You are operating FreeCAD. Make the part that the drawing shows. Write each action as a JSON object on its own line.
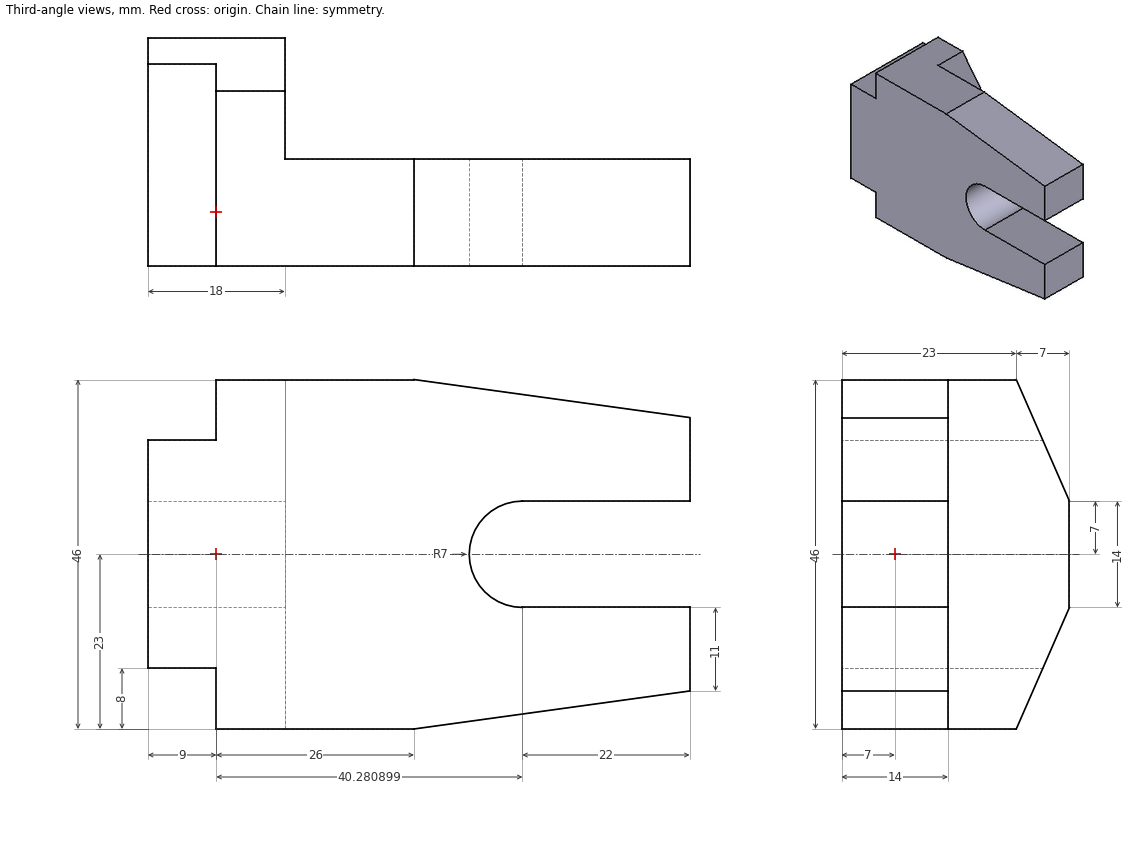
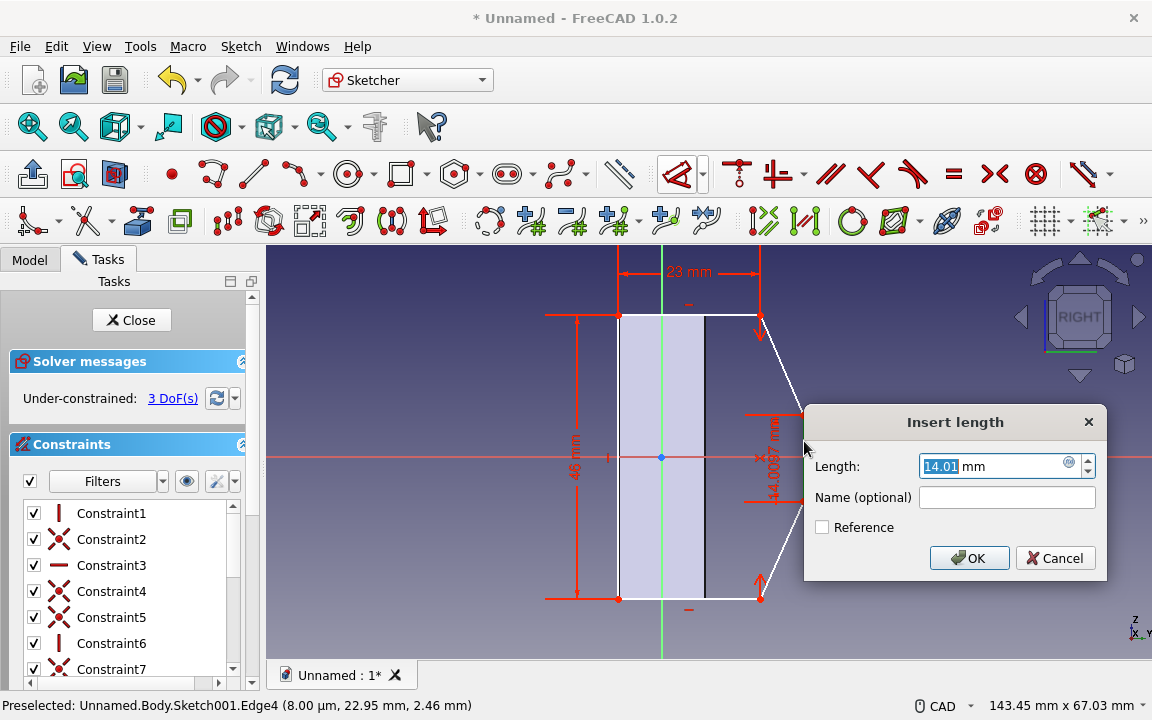
{"action": "type", "text": "14"}
{"action": "key", "text": "Return"}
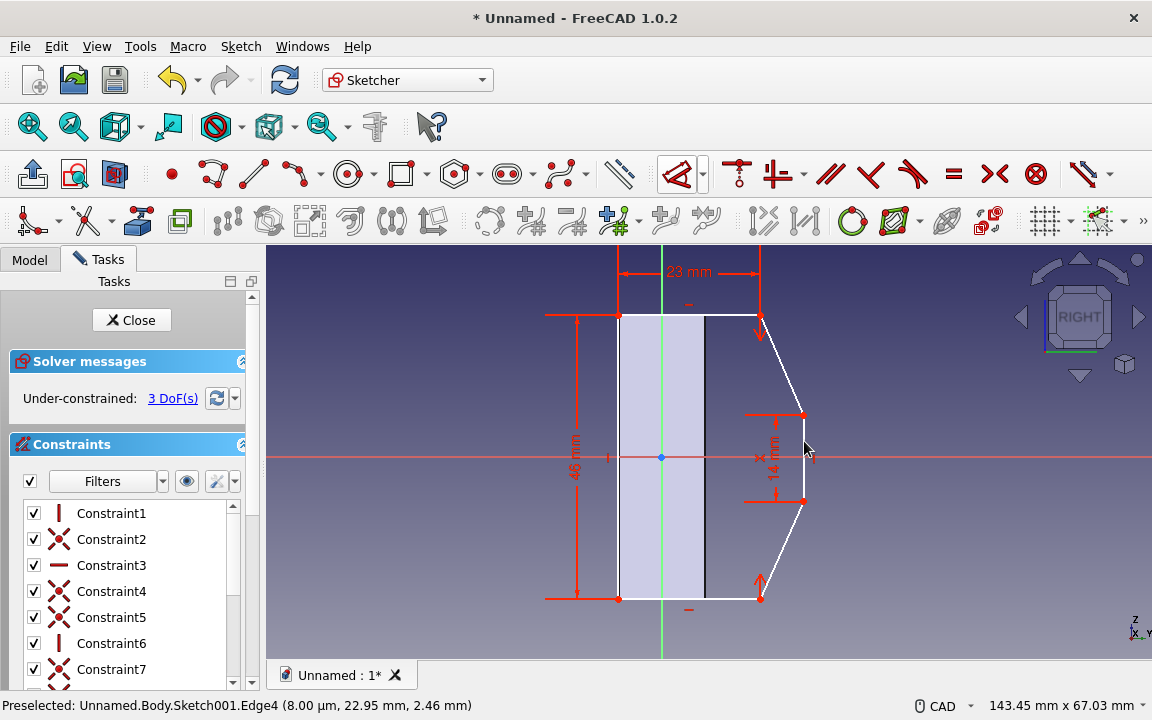
{"action": "left_click", "coordinate": [618, 599]}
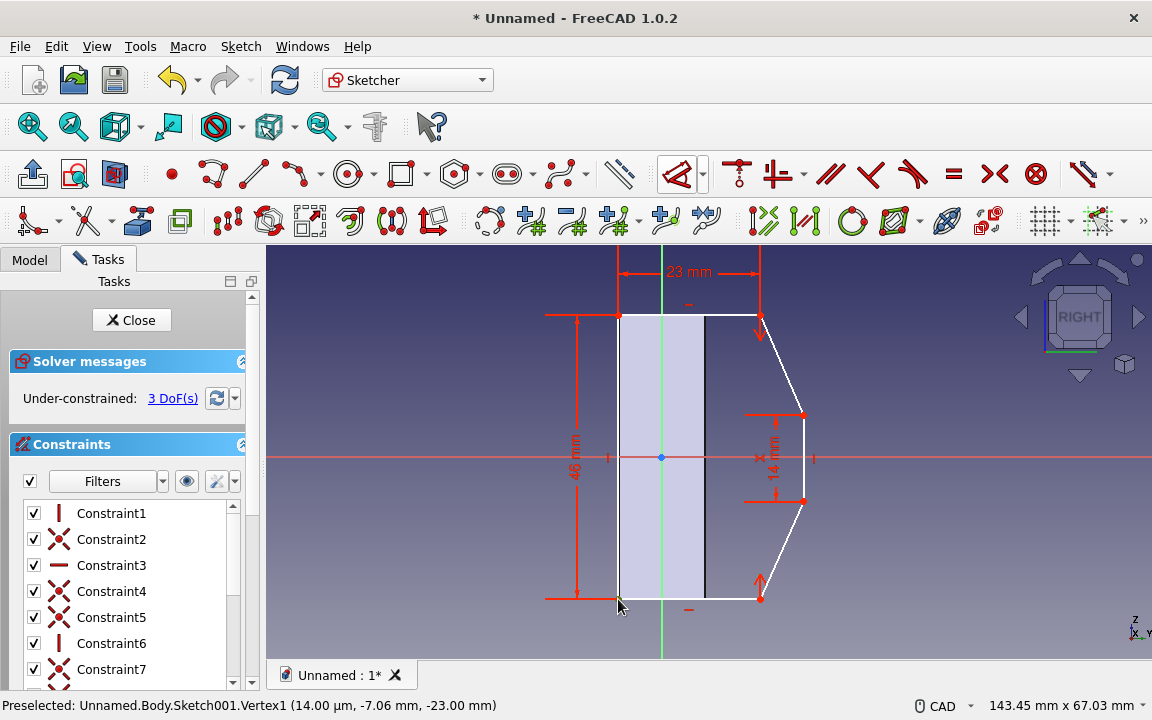
{"action": "key", "text": "l"}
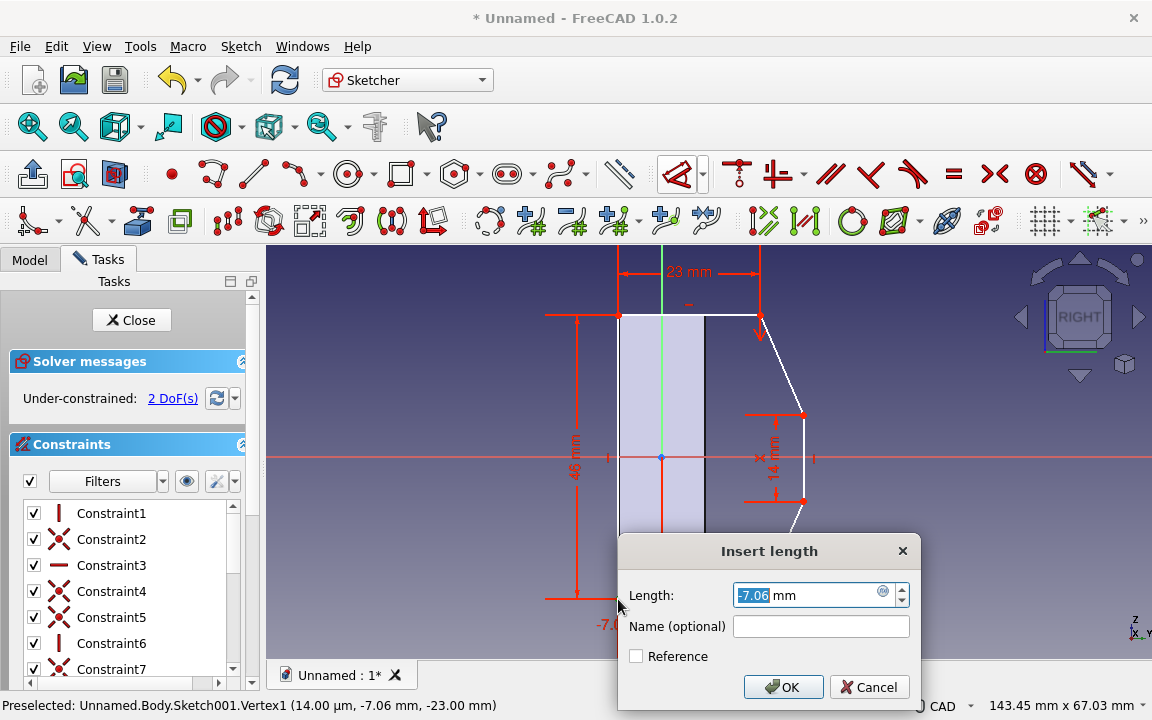
{"action": "type", "text": "-7"}
{"action": "key", "text": "Return"}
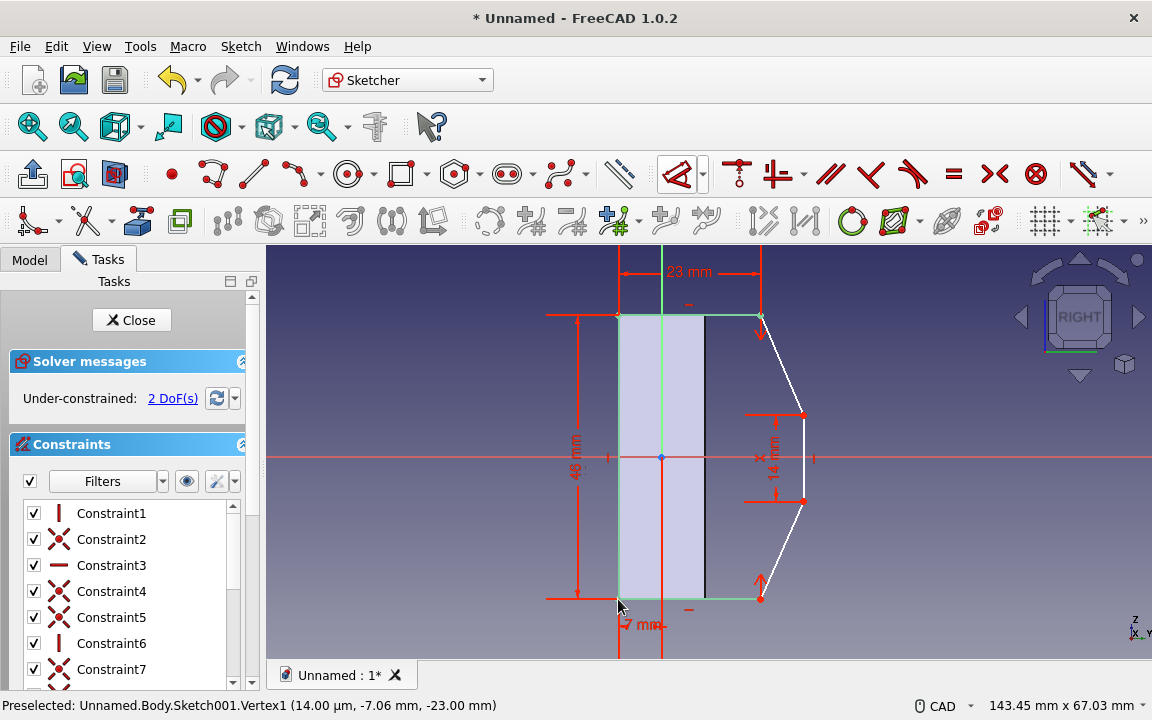
{"action": "left_click", "coordinate": [804, 415]}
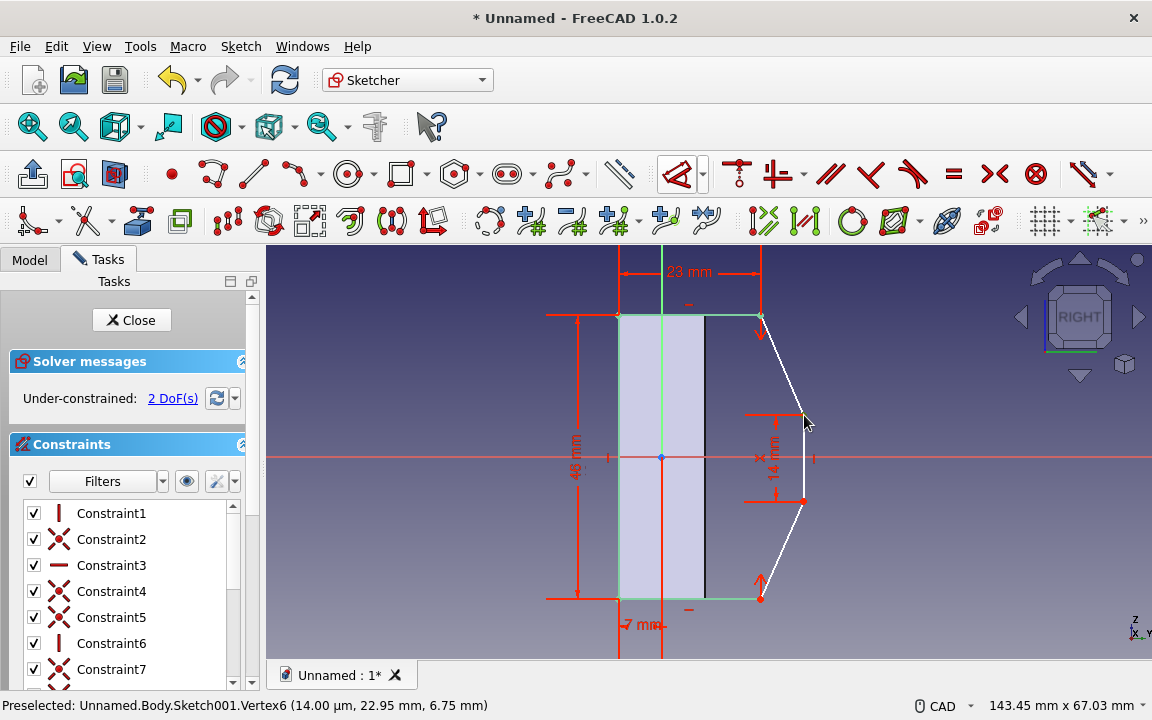
{"action": "key", "text": "i"}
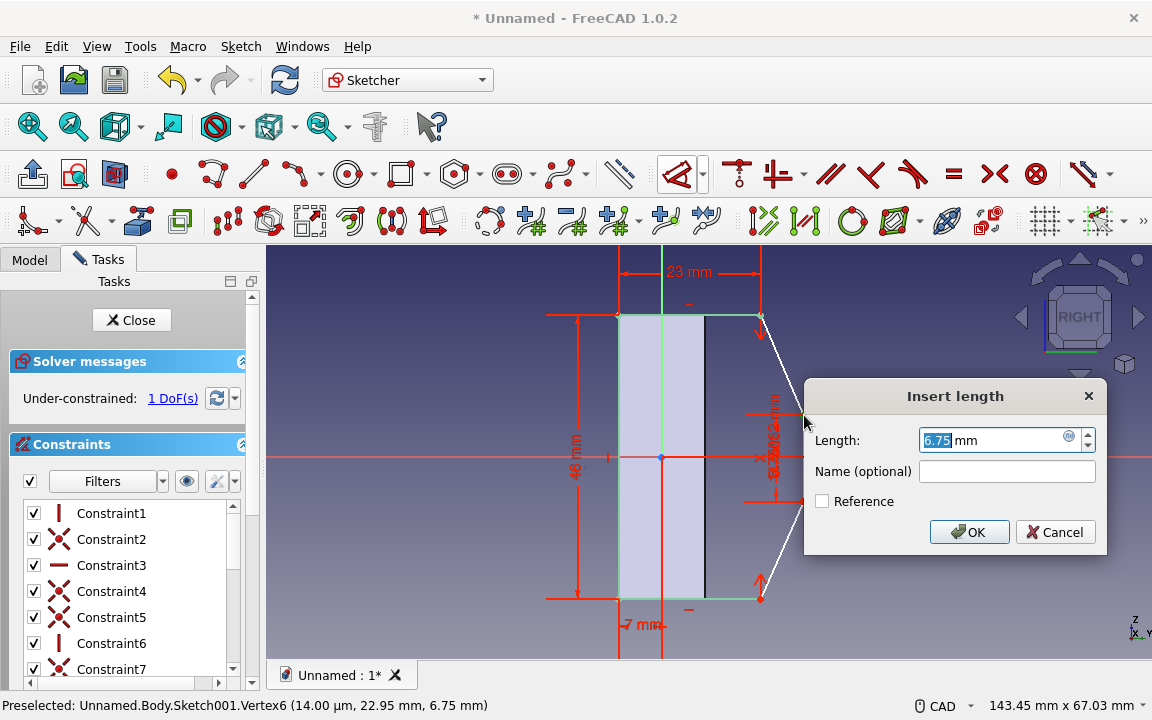
{"action": "type", "text": "7"}
{"action": "key", "text": "Return"}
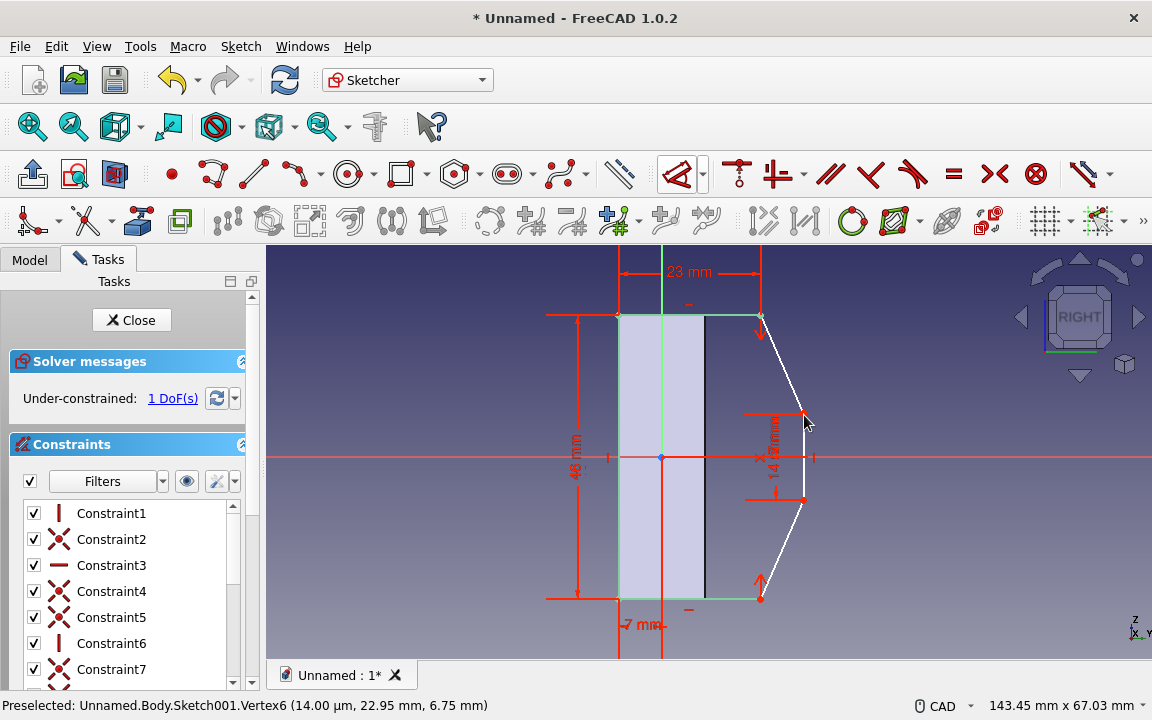
{"action": "left_click", "coordinate": [774, 345]}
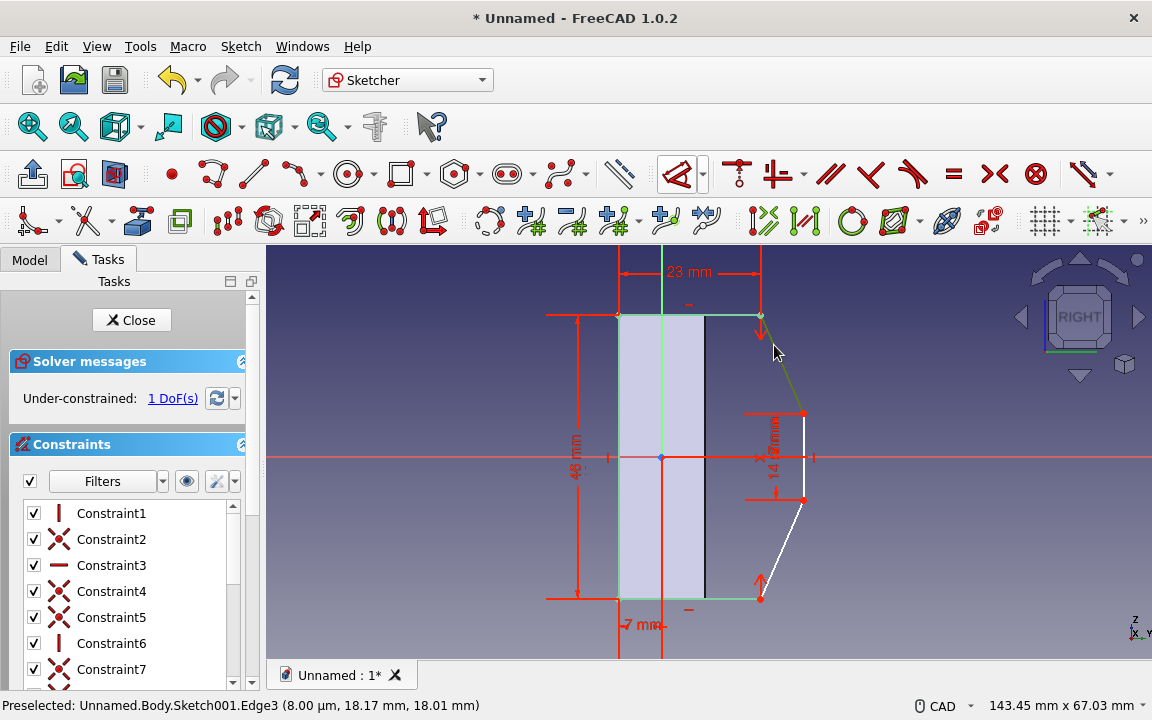
{"action": "key", "text": "l"}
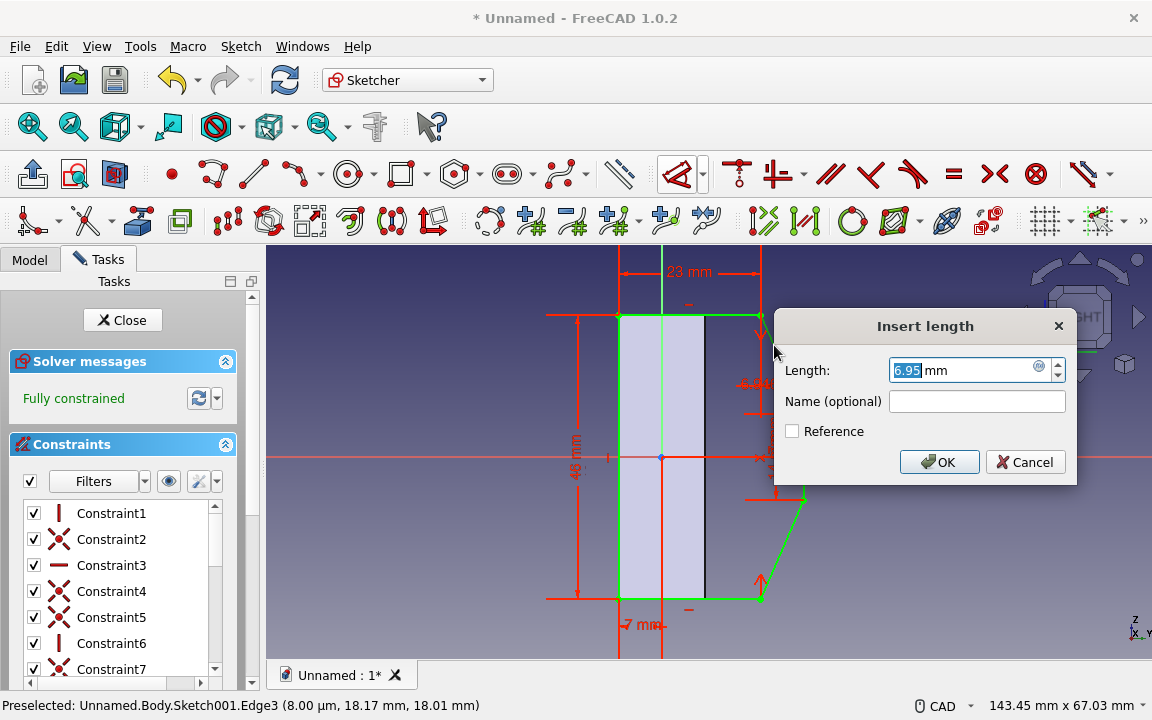
{"action": "type", "text": "7"}
{"action": "key", "text": "Return"}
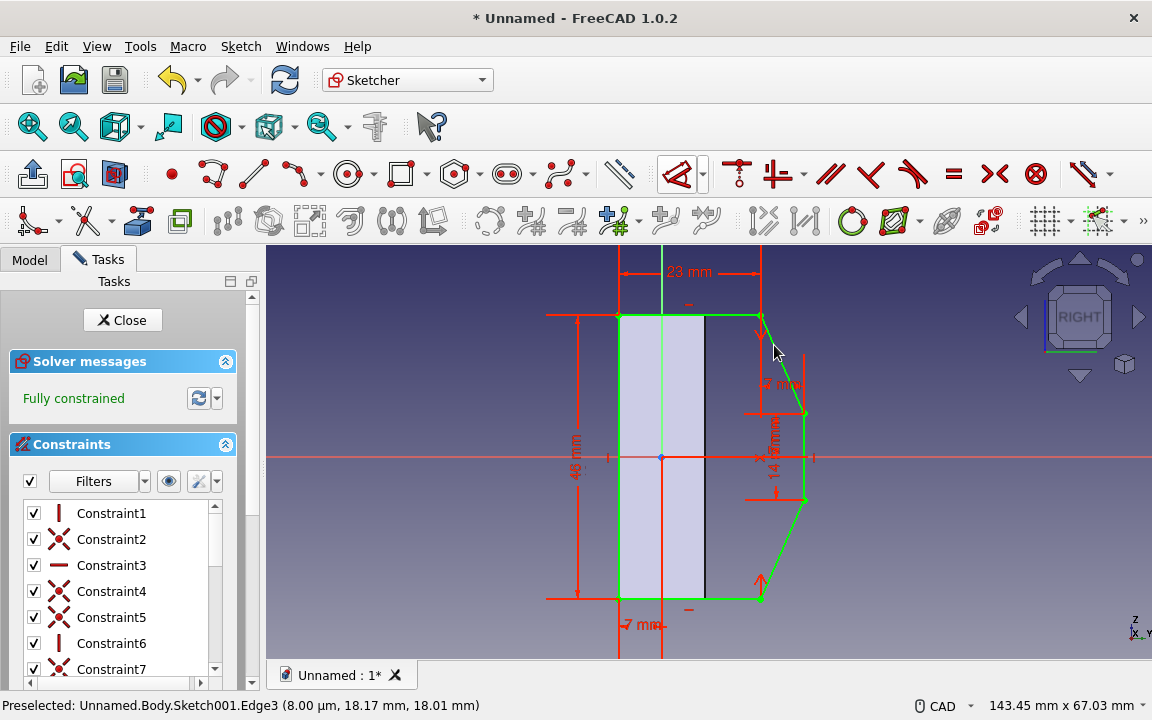
{"action": "left_click", "coordinate": [123, 320]}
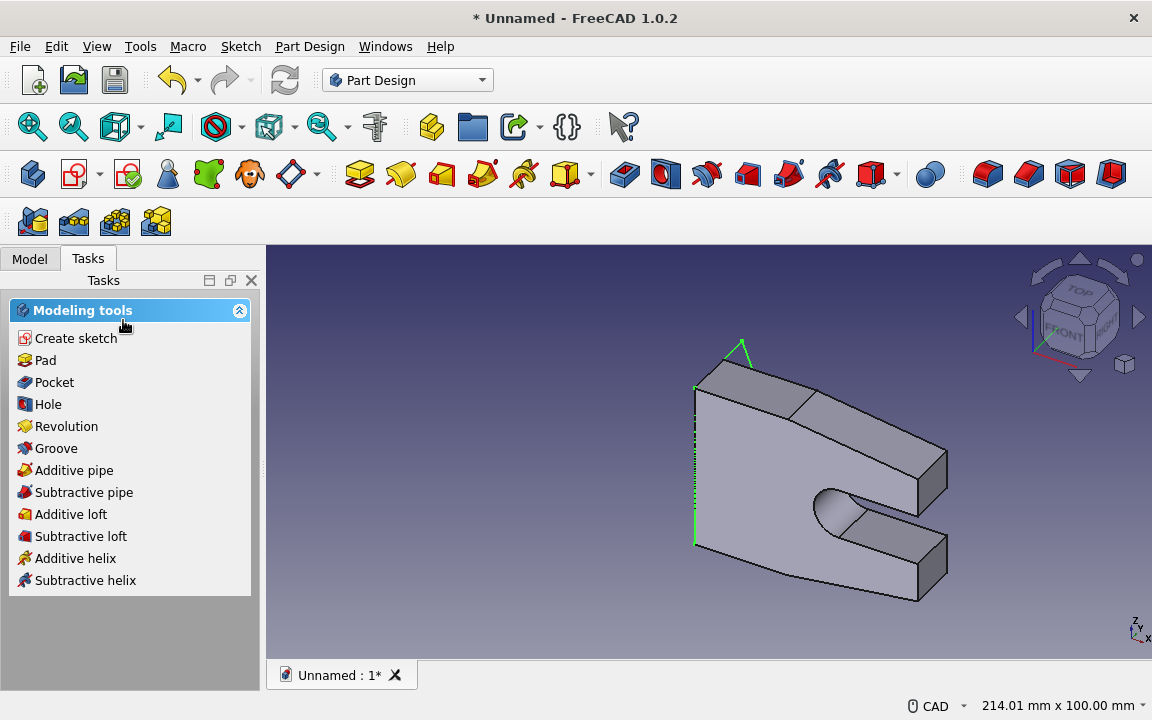
{"action": "left_click", "coordinate": [360, 174]}